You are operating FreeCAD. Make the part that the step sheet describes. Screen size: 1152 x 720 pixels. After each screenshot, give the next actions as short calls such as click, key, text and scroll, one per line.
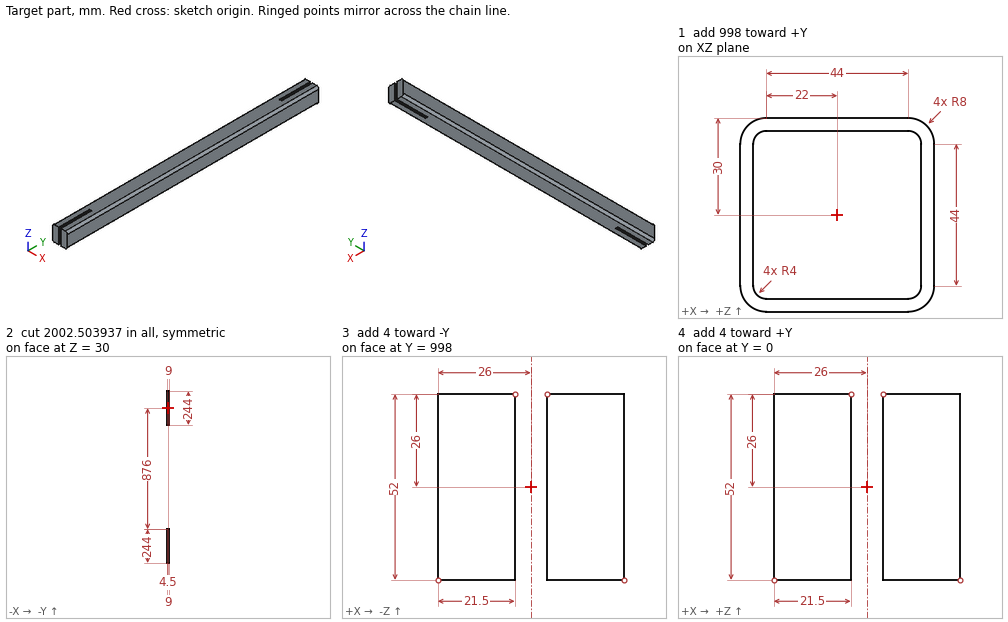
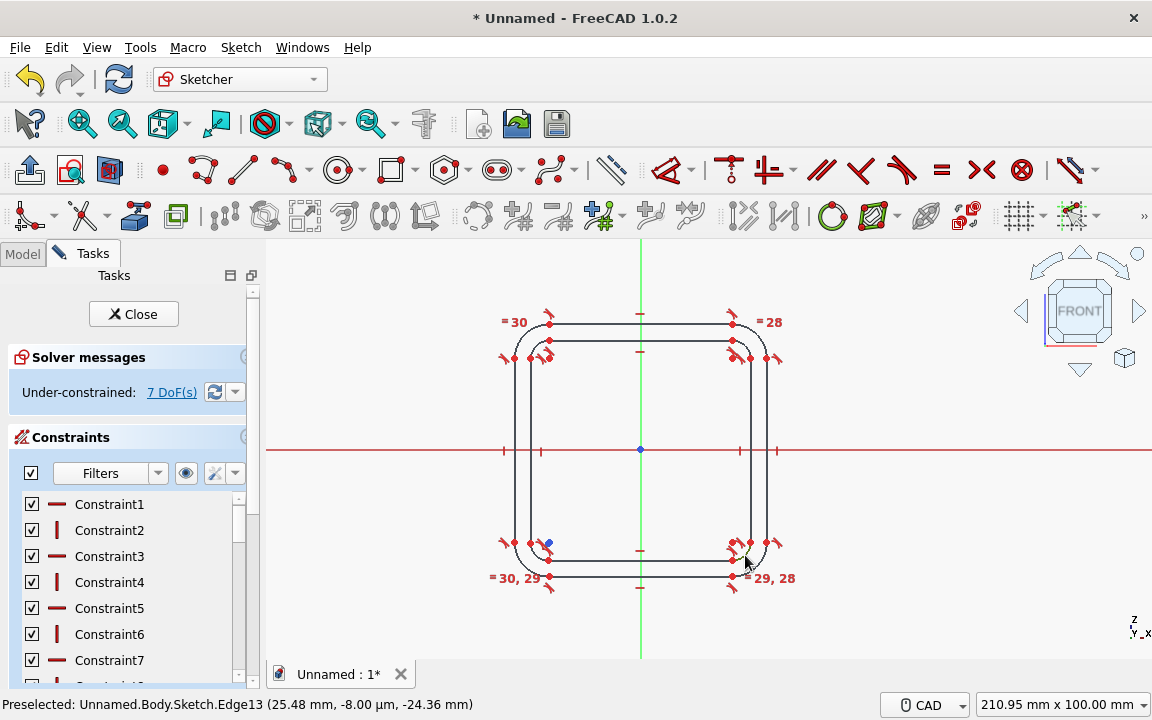
click(536, 556)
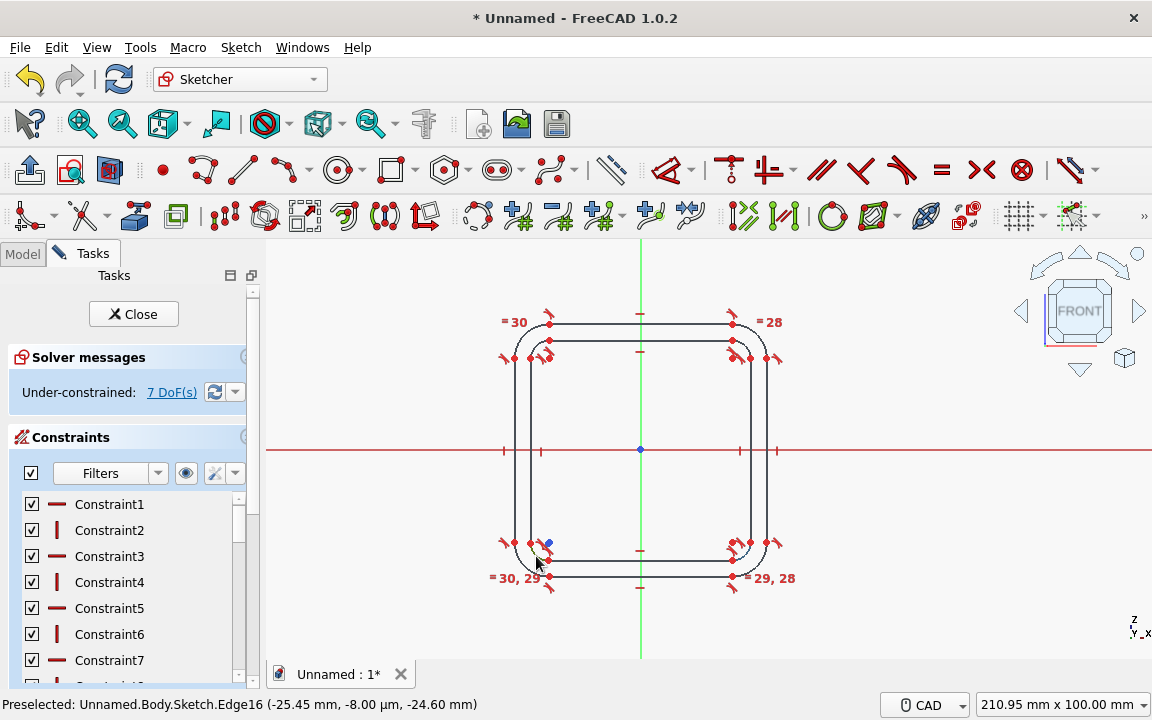
click(942, 170)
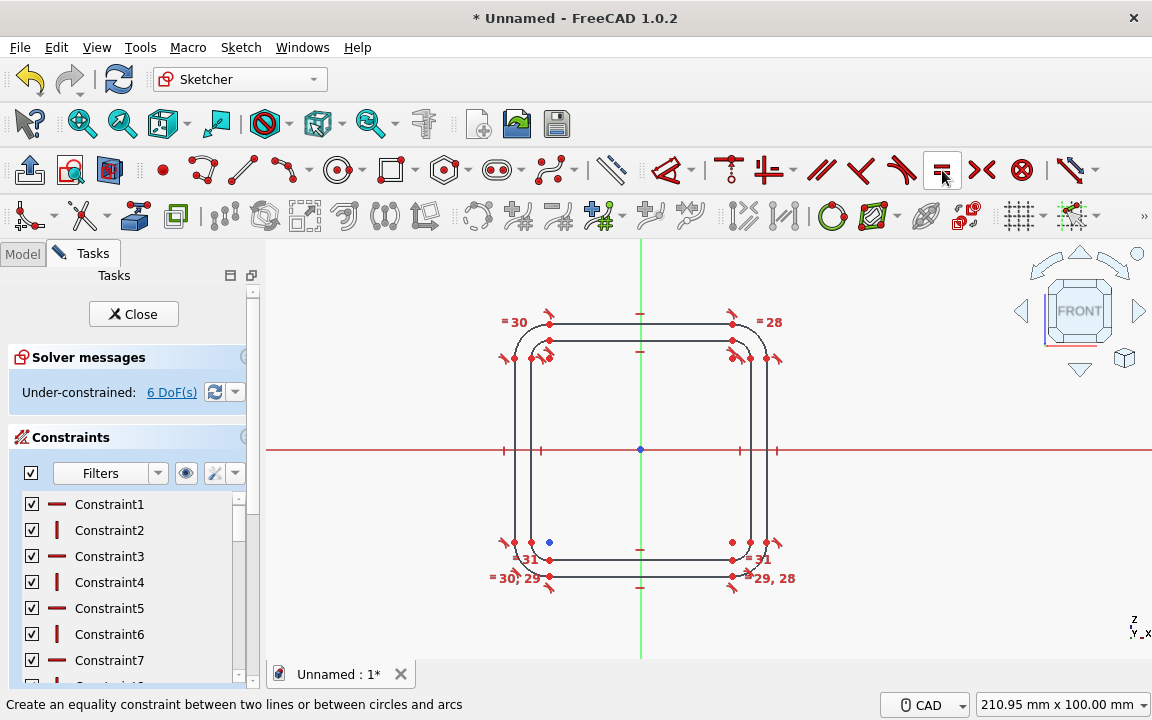
click(666, 170)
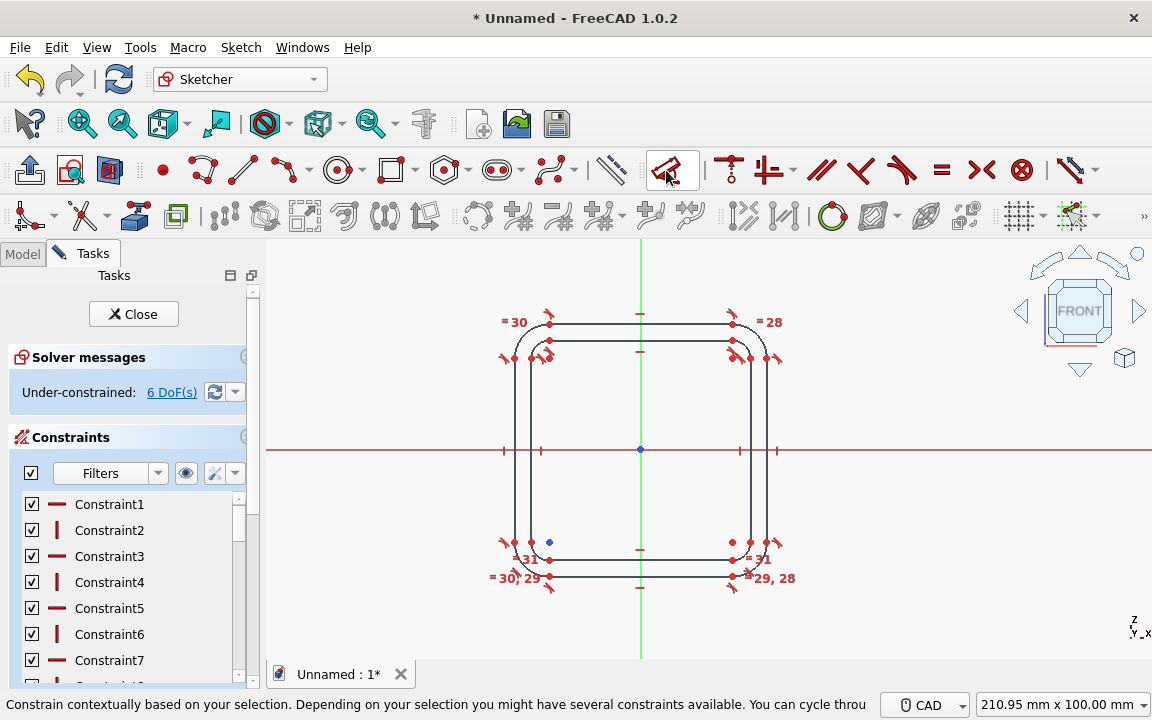
click(763, 343)
click(791, 328)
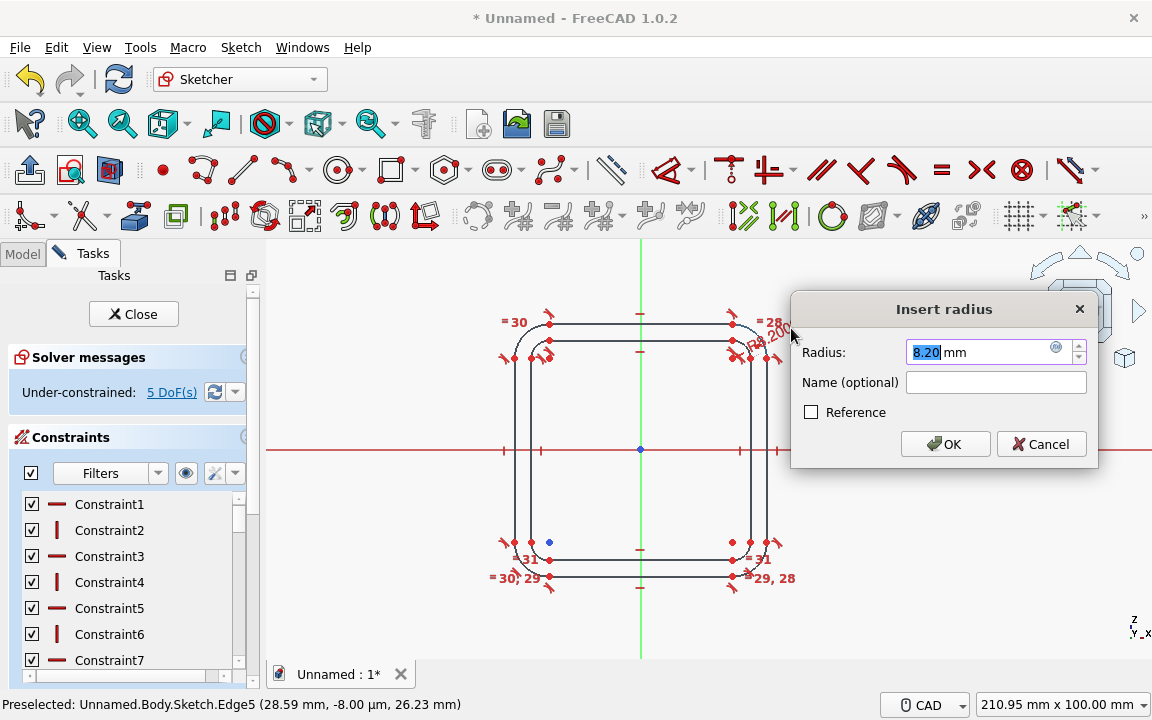
text(8)
key(Return)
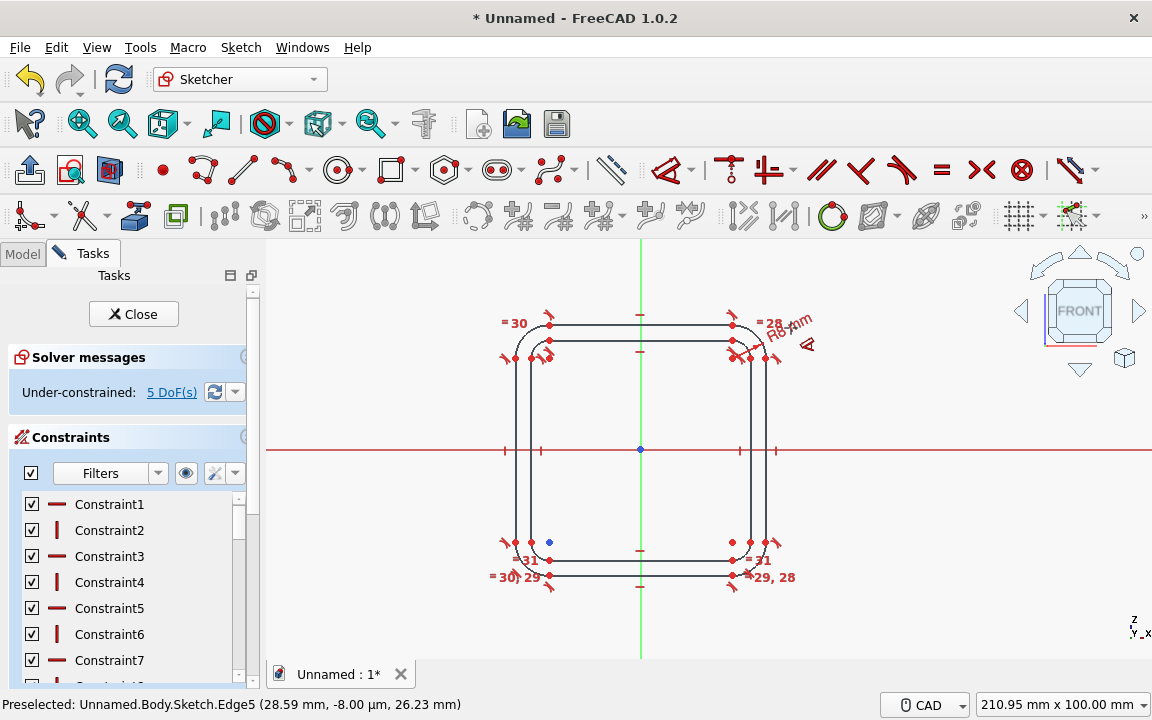
scroll(745, 555, up, 5)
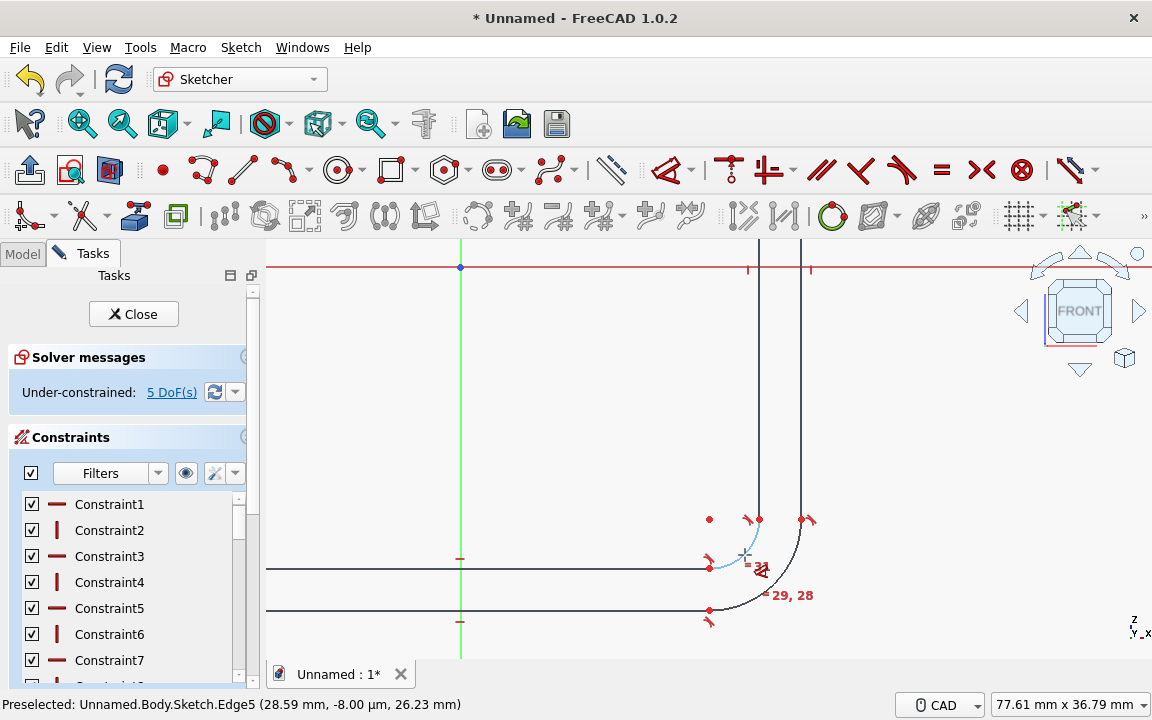
click(745, 554)
click(652, 462)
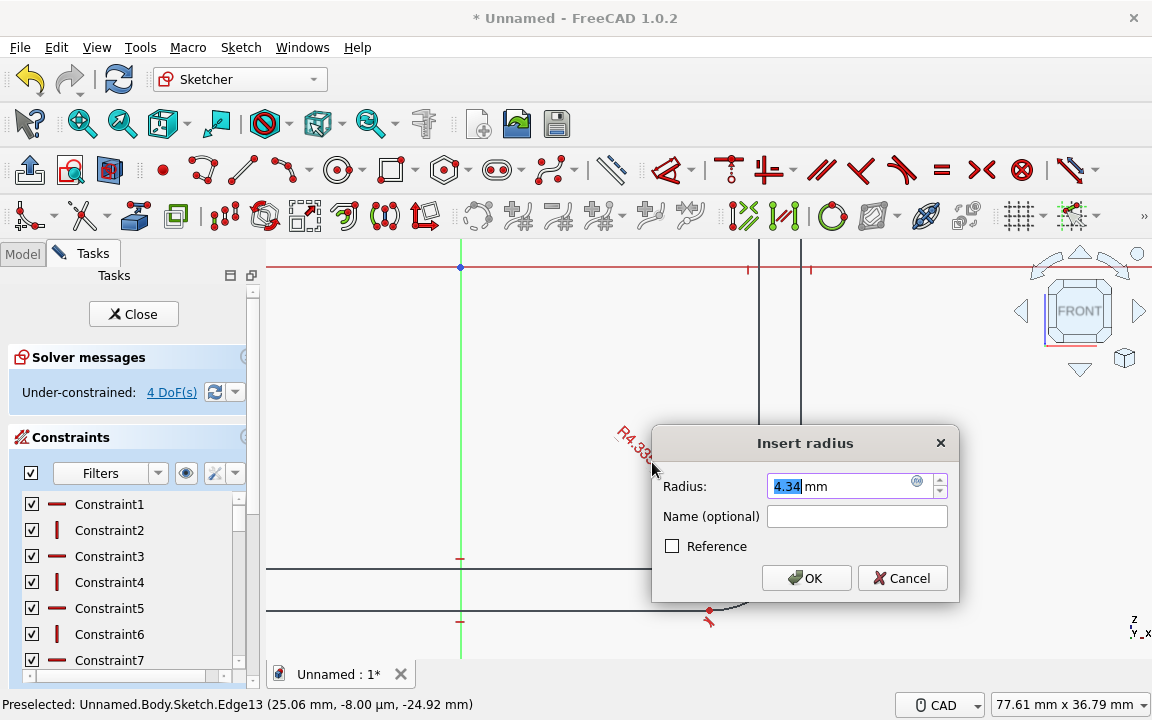
text(4)
key(Return)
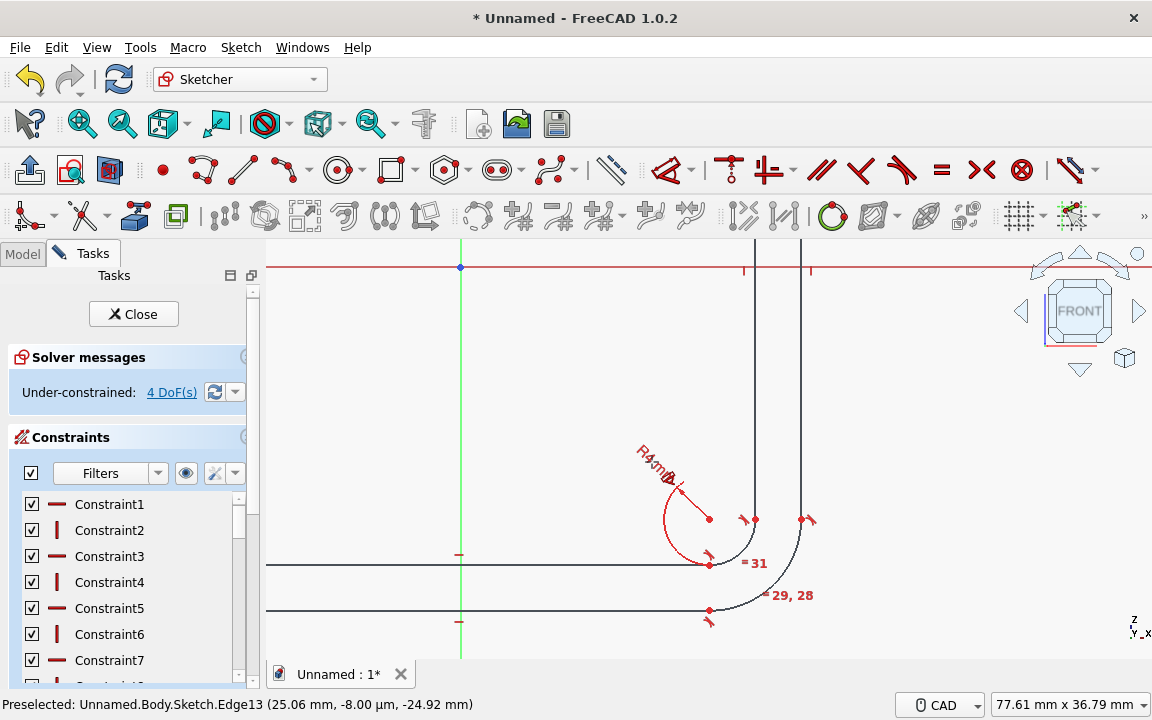
scroll(745, 555, down, 5)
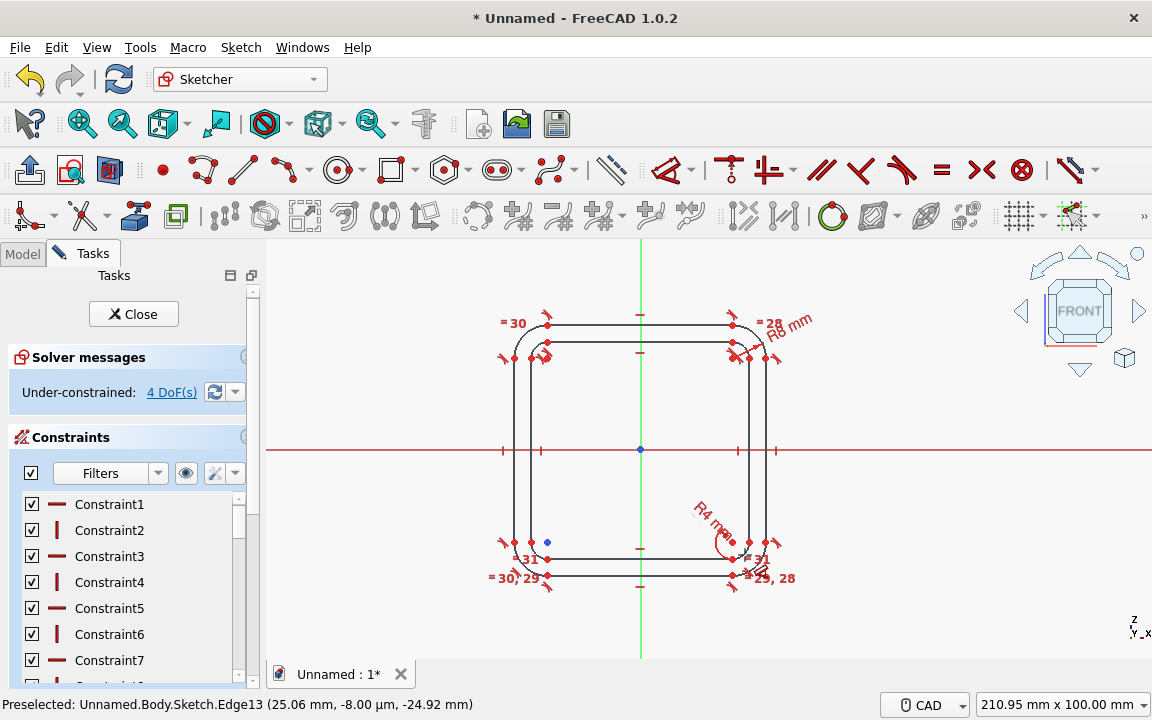
click(603, 325)
click(598, 291)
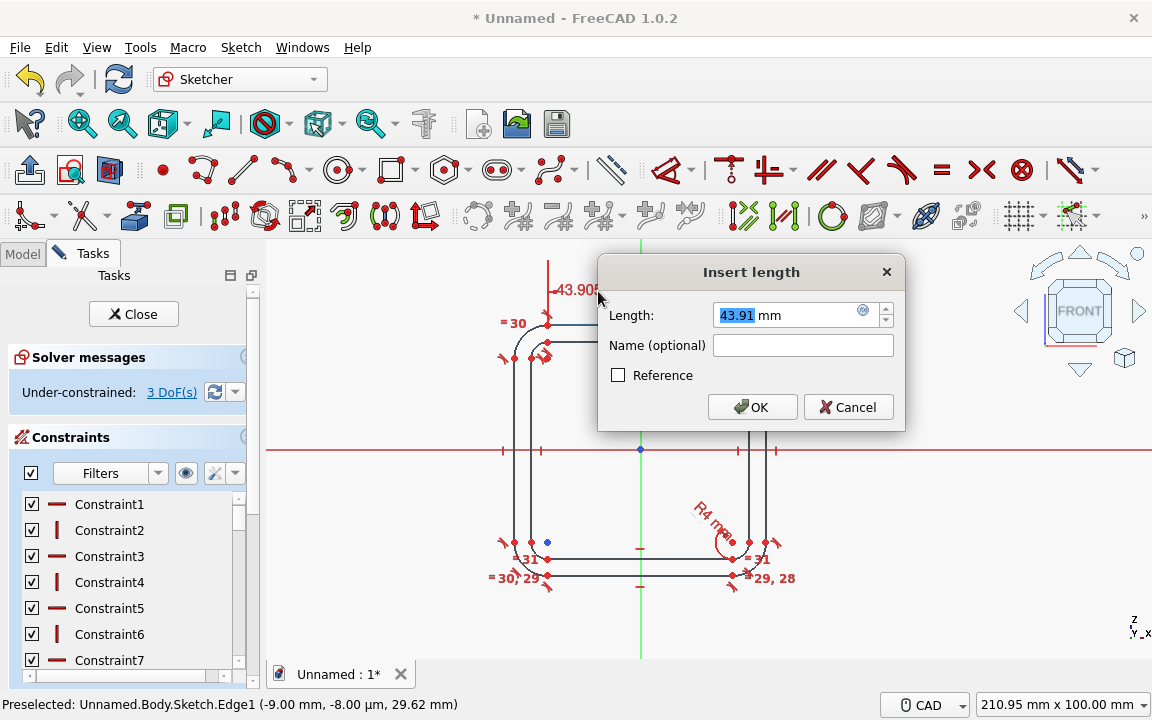
text(44)
key(Return)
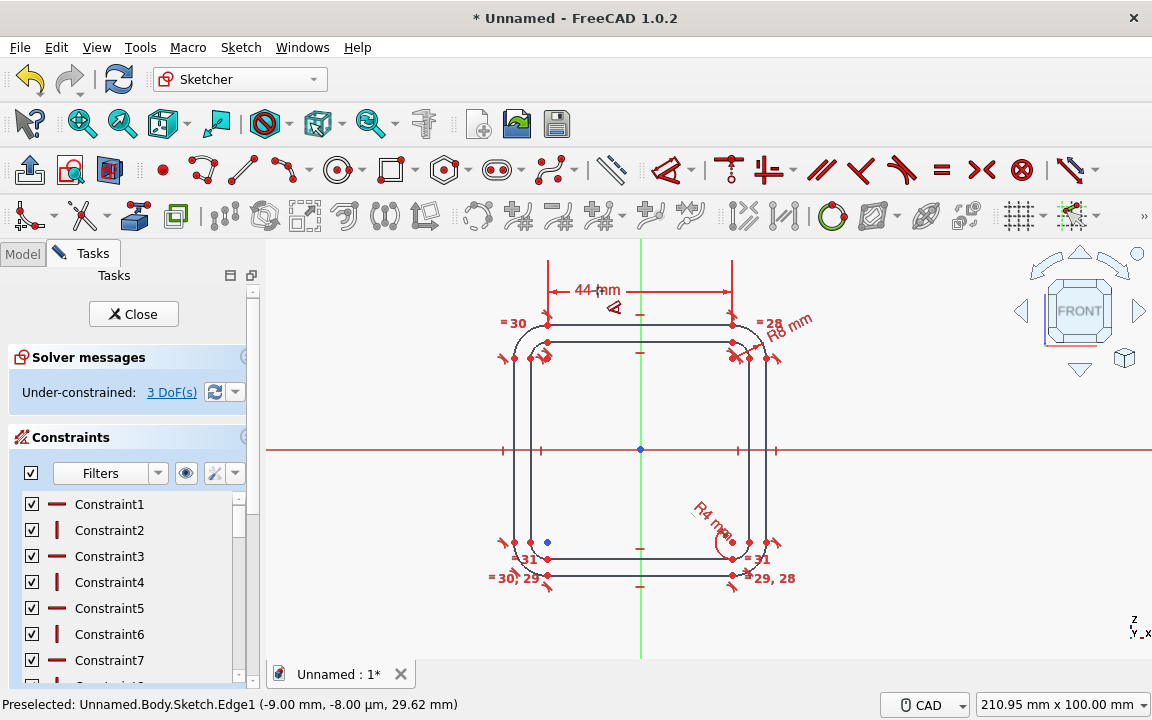
click(766, 414)
click(800, 408)